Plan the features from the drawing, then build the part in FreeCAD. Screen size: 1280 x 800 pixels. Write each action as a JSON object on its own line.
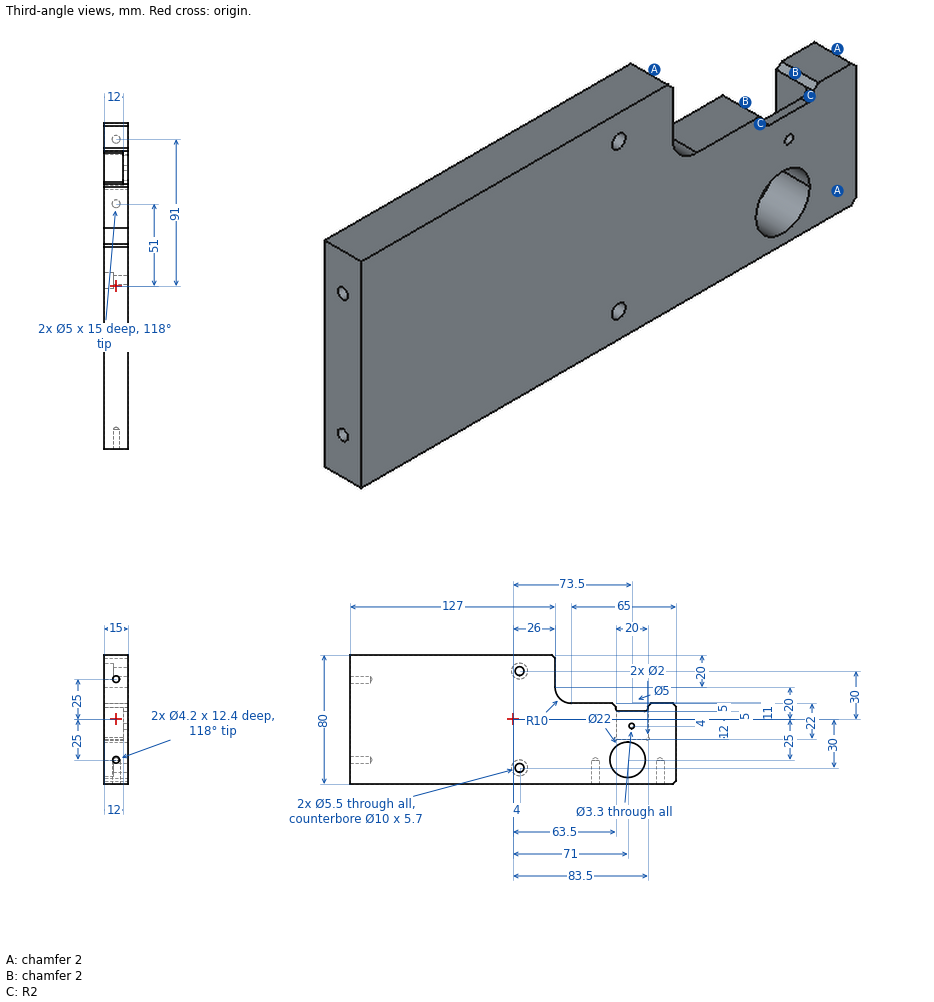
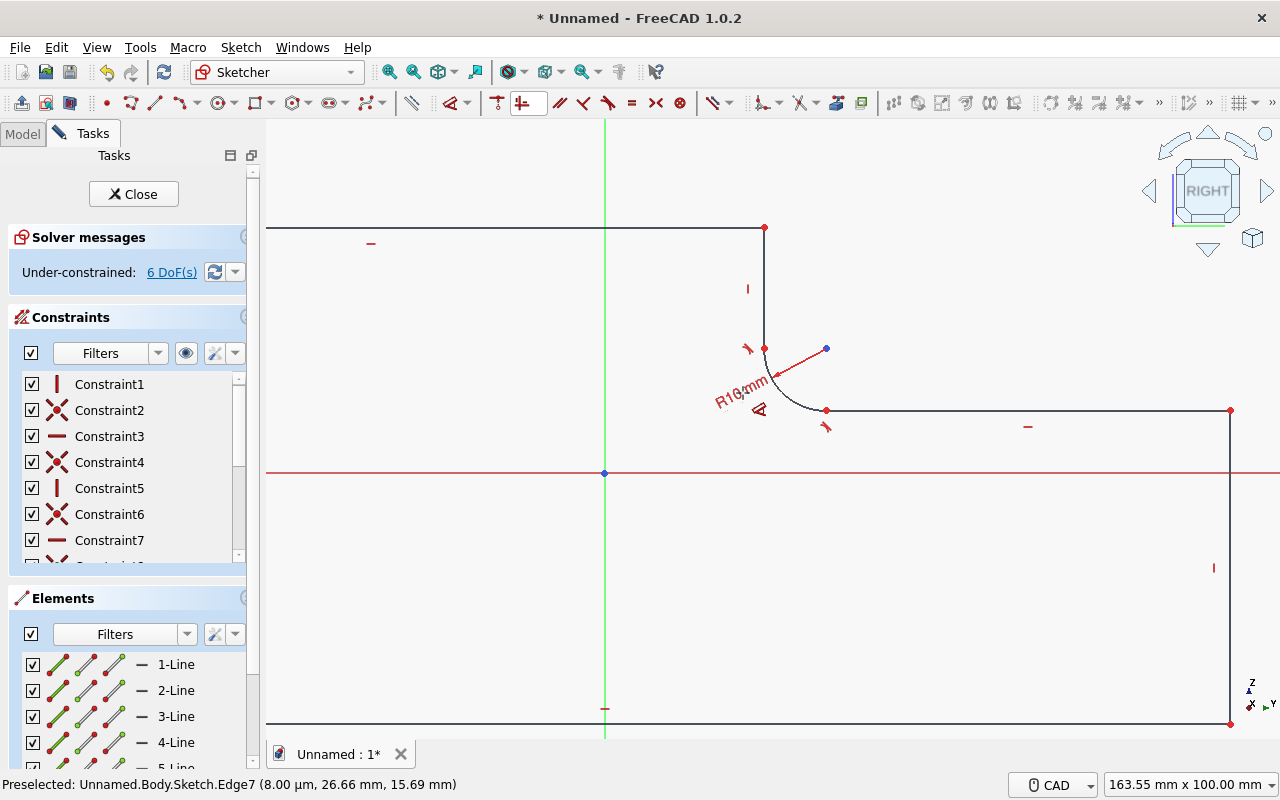
{"action": "left_click", "coordinate": [764, 313]}
{"action": "left_click", "coordinate": [798, 288]}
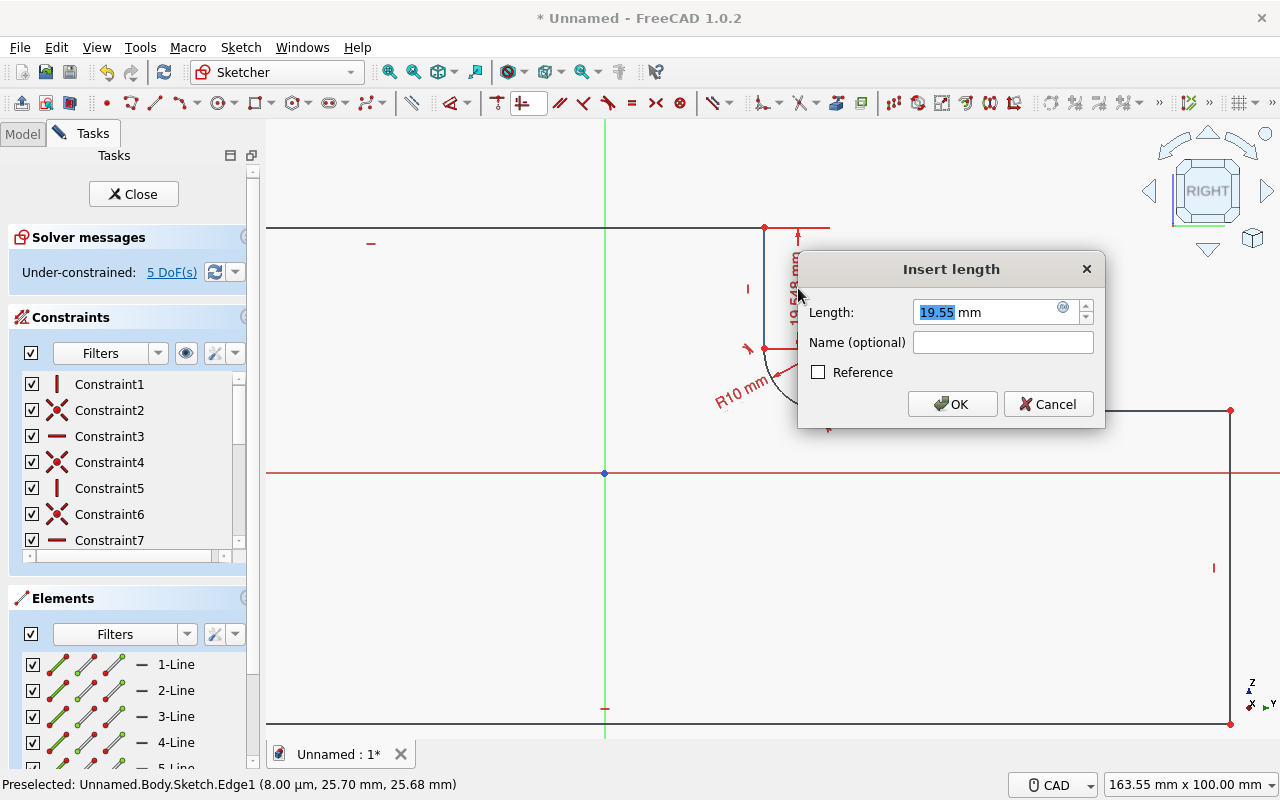
{"action": "type", "text": "20"}
{"action": "key", "text": "Return"}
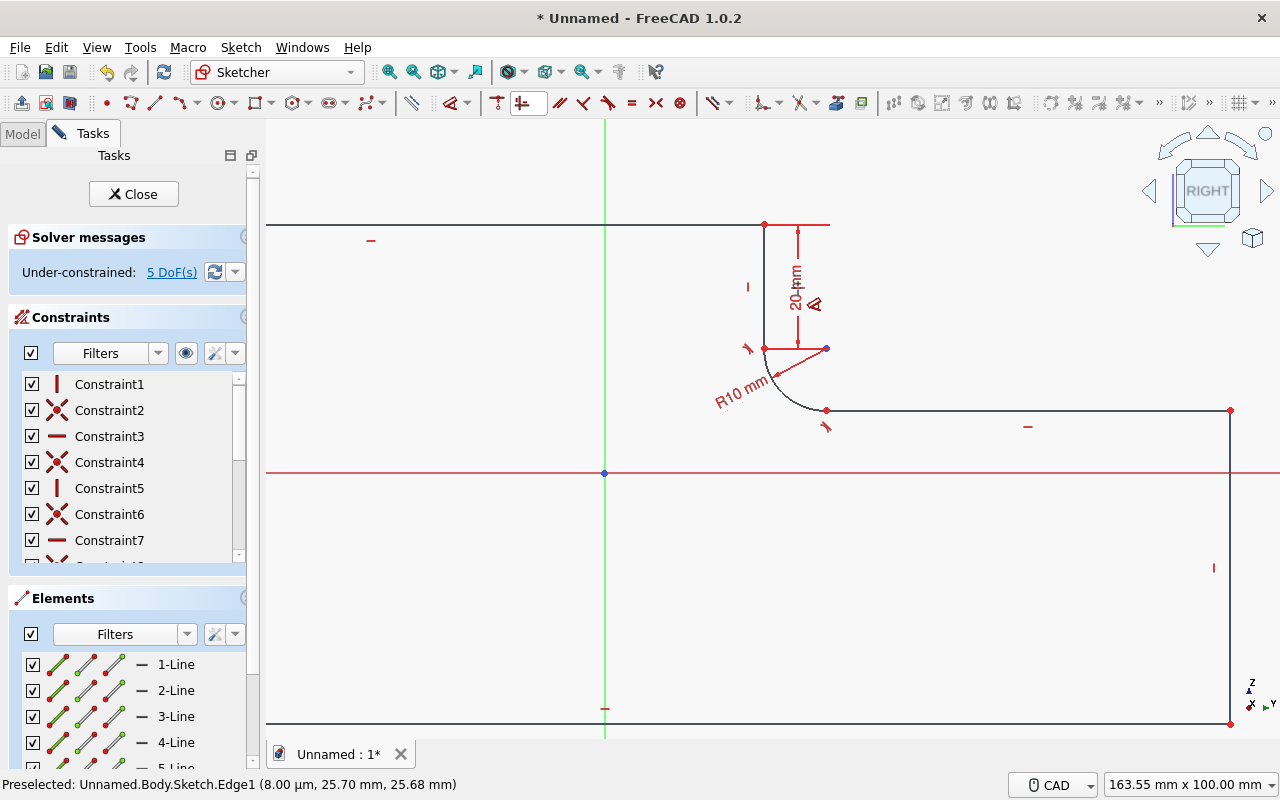
{"action": "scroll", "coordinate": [786, 393], "scroll_direction": "down", "scroll_amount": 4}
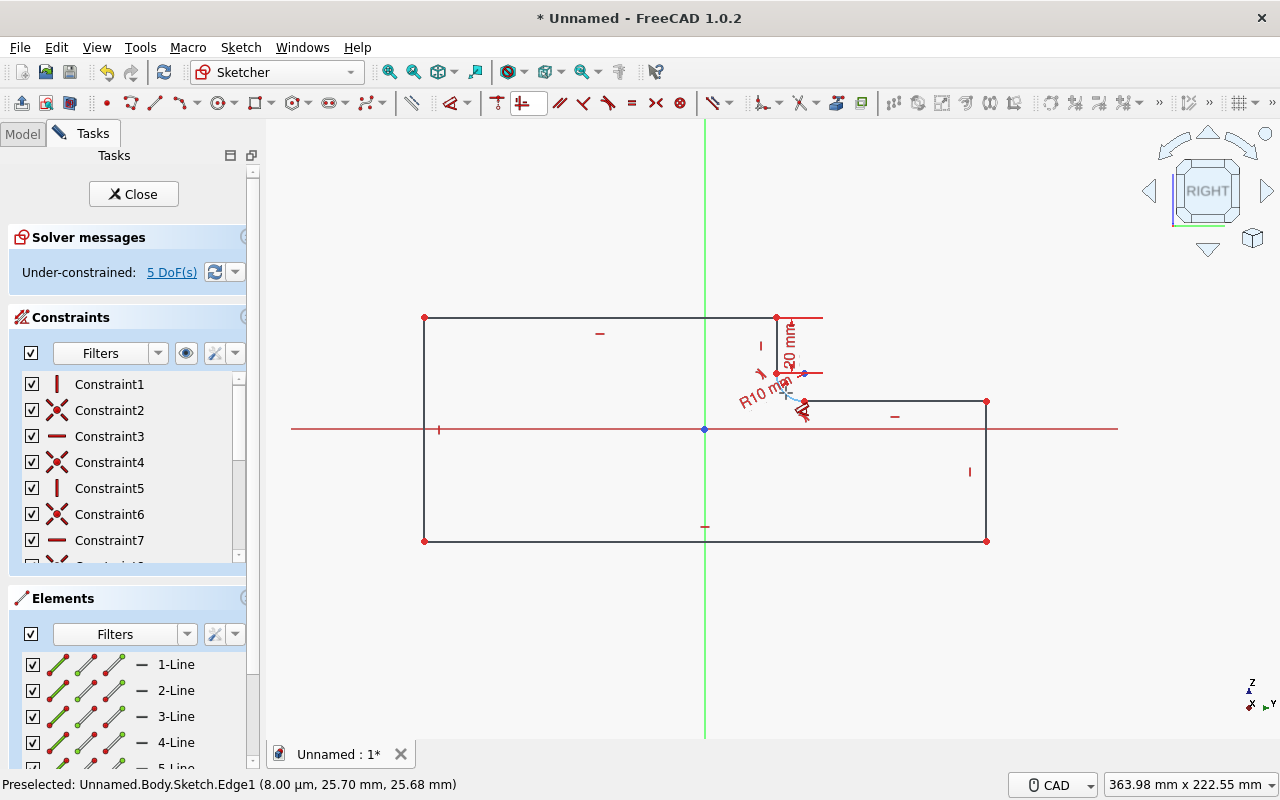
{"action": "left_click", "coordinate": [424, 385]}
{"action": "left_click", "coordinate": [390, 378]}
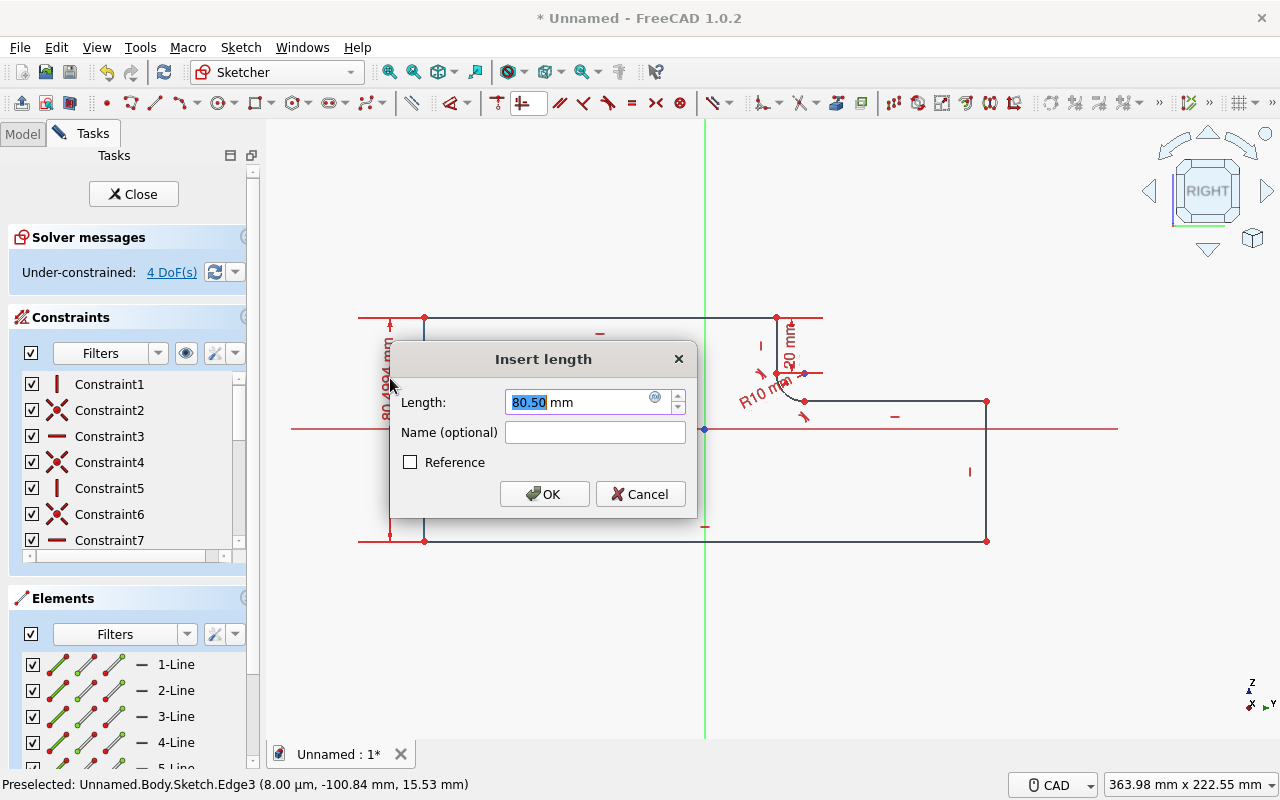
{"action": "type", "text": "80"}
{"action": "key", "text": "Return"}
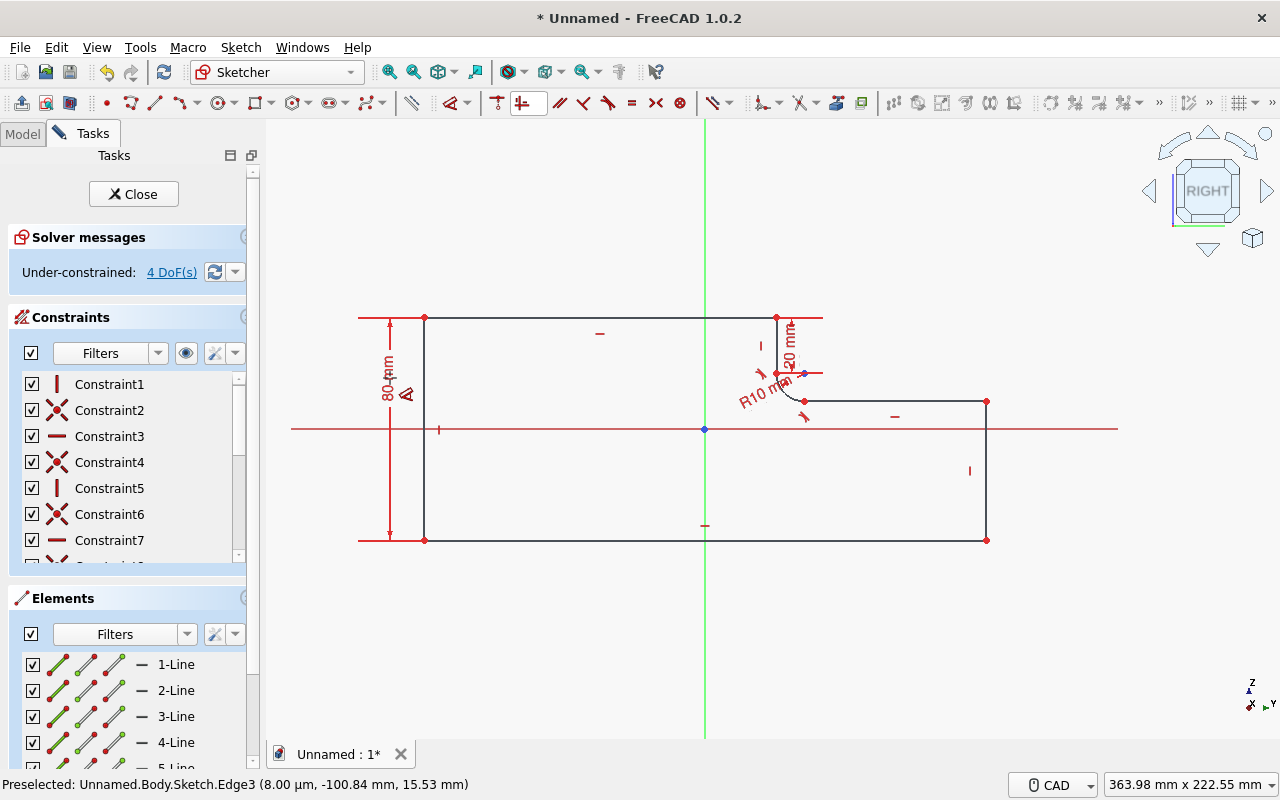
{"action": "left_click", "coordinate": [932, 401]}
{"action": "left_click", "coordinate": [895, 367]}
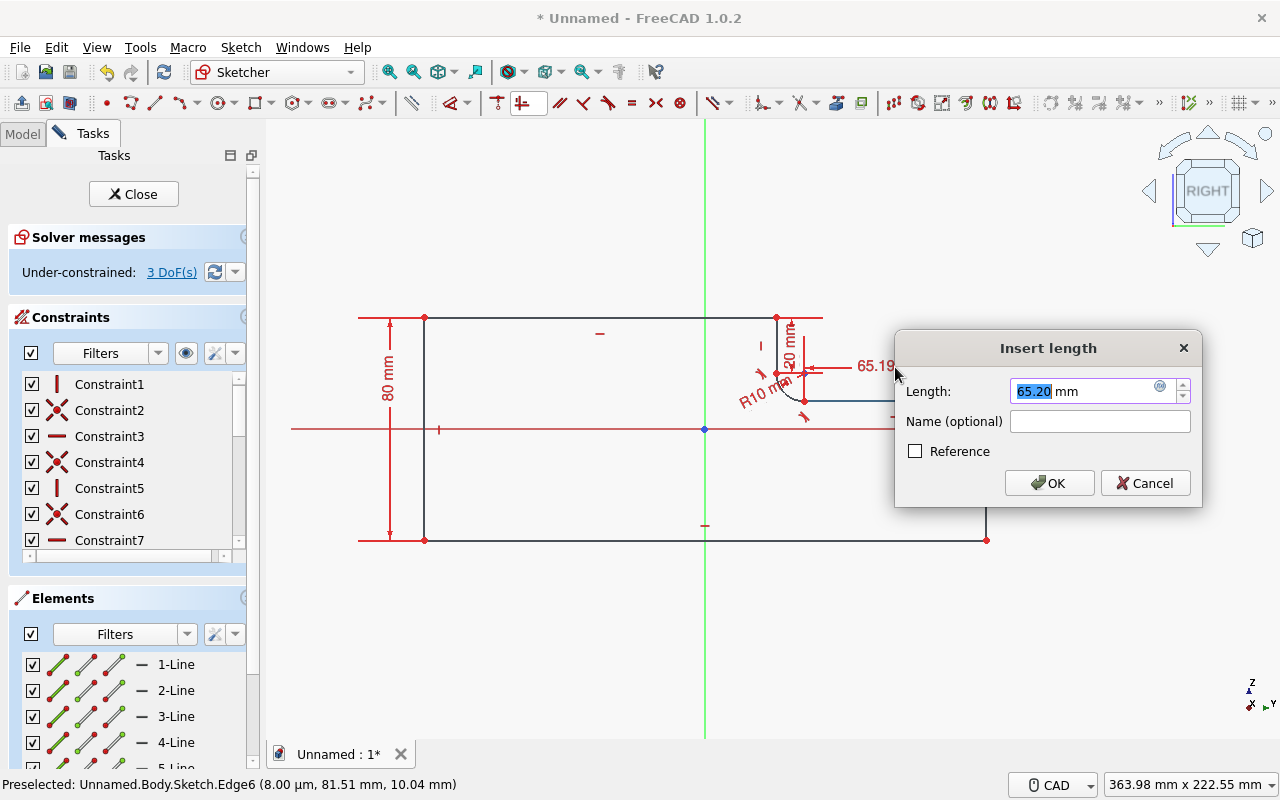
{"action": "type", "text": "65"}
{"action": "key", "text": "Return"}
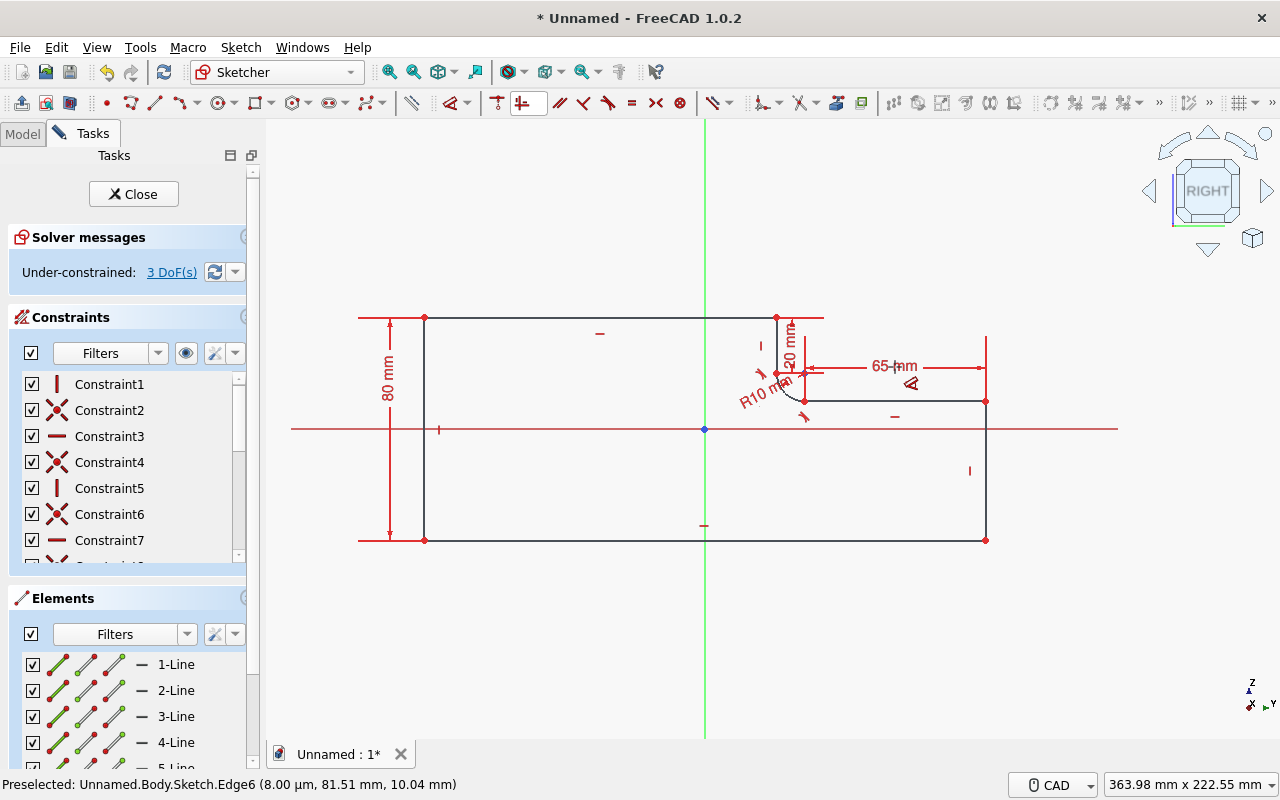
{"action": "left_click", "coordinate": [671, 318]}
{"action": "left_click", "coordinate": [600, 284]}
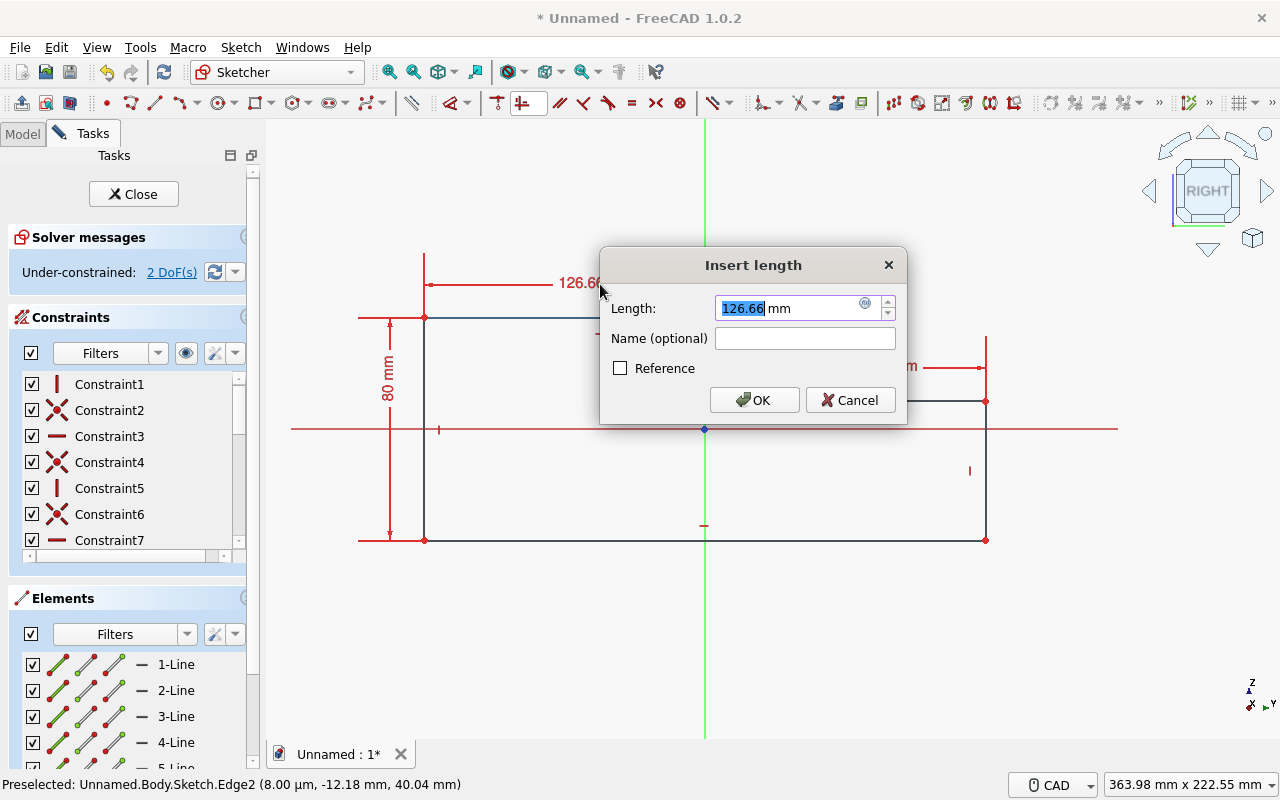
{"action": "type", "text": "127"}
{"action": "key", "text": "Return"}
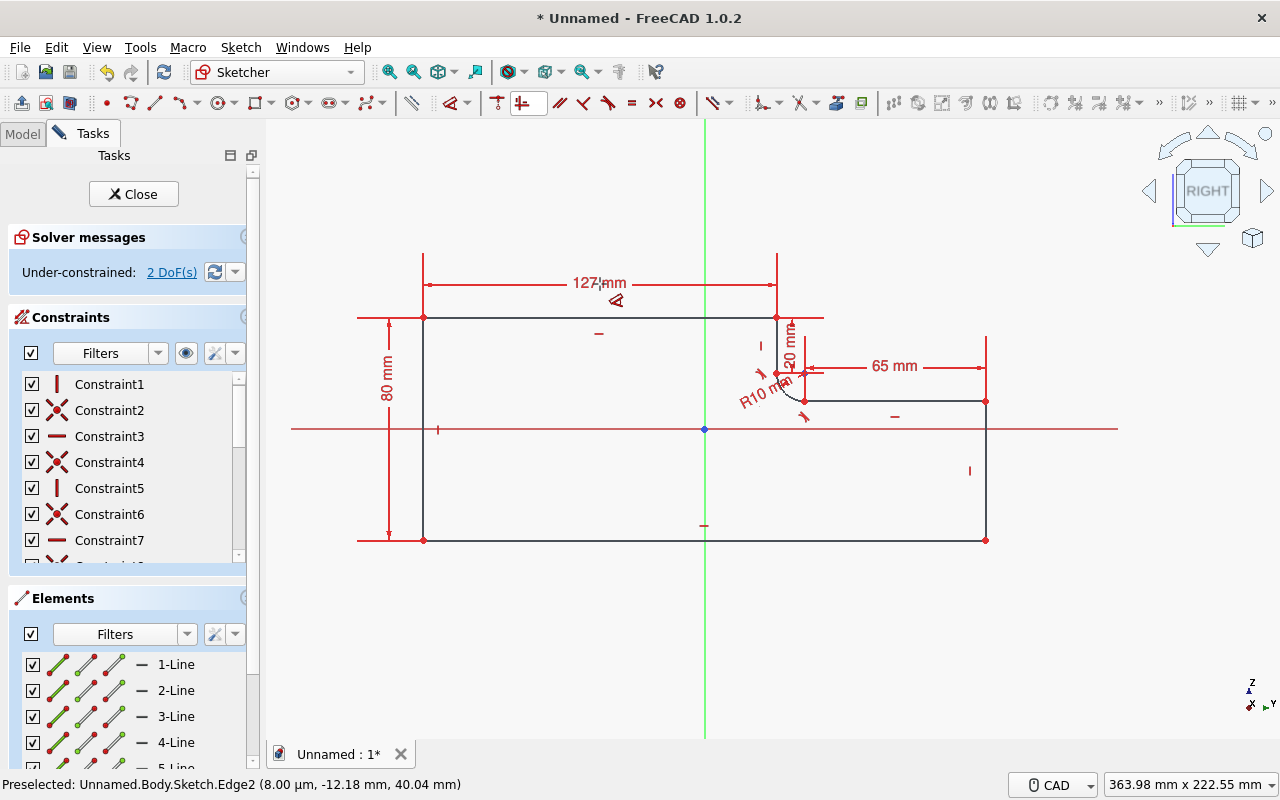
{"action": "left_click", "coordinate": [777, 373]}
{"action": "left_click", "coordinate": [741, 463]}